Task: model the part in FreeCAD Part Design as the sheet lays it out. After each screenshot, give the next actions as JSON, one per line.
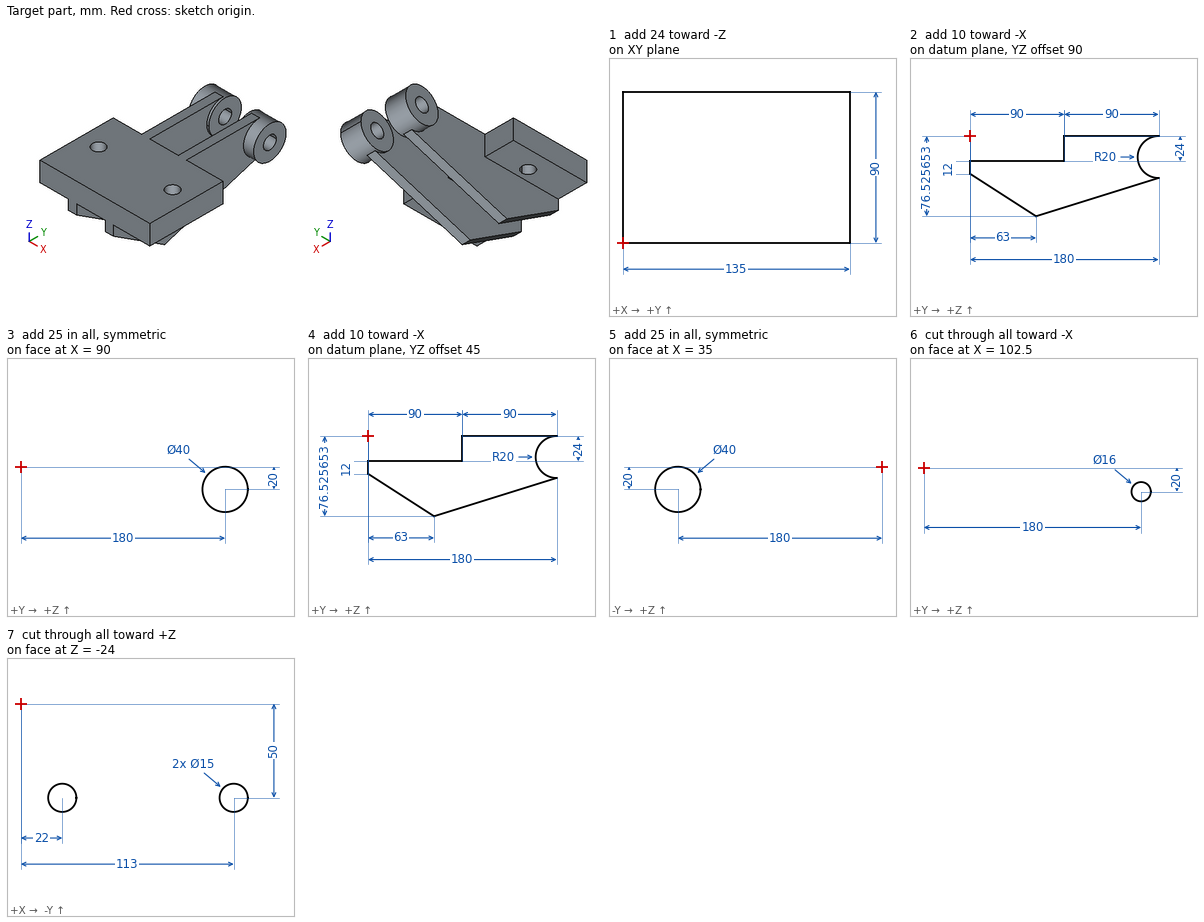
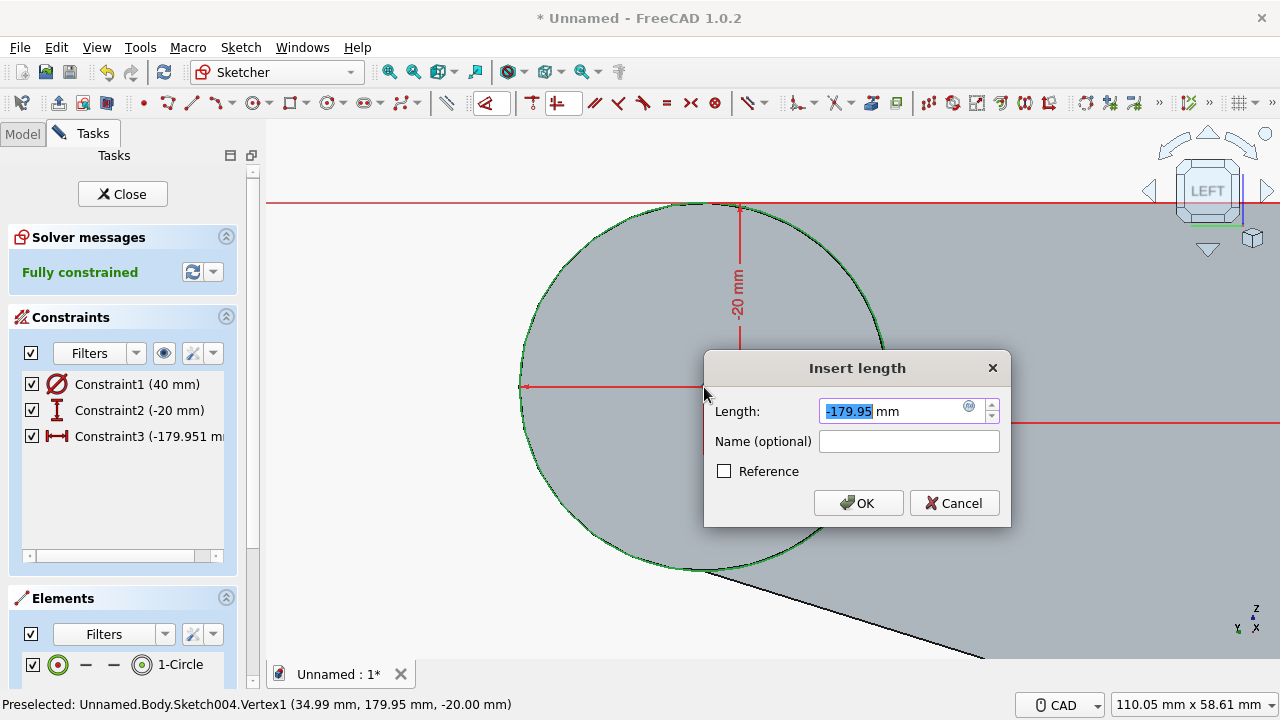
{"action": "type", "text": "-180"}
{"action": "key", "text": "Return"}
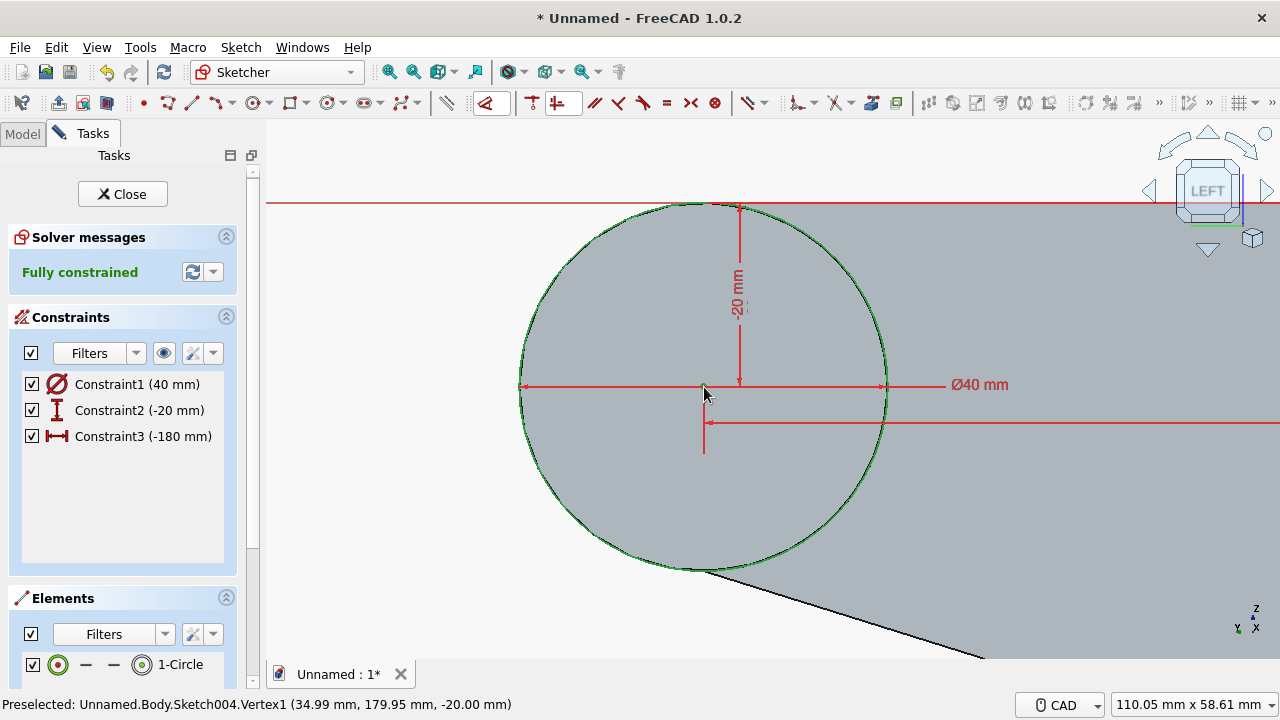
{"action": "left_click", "coordinate": [123, 194]}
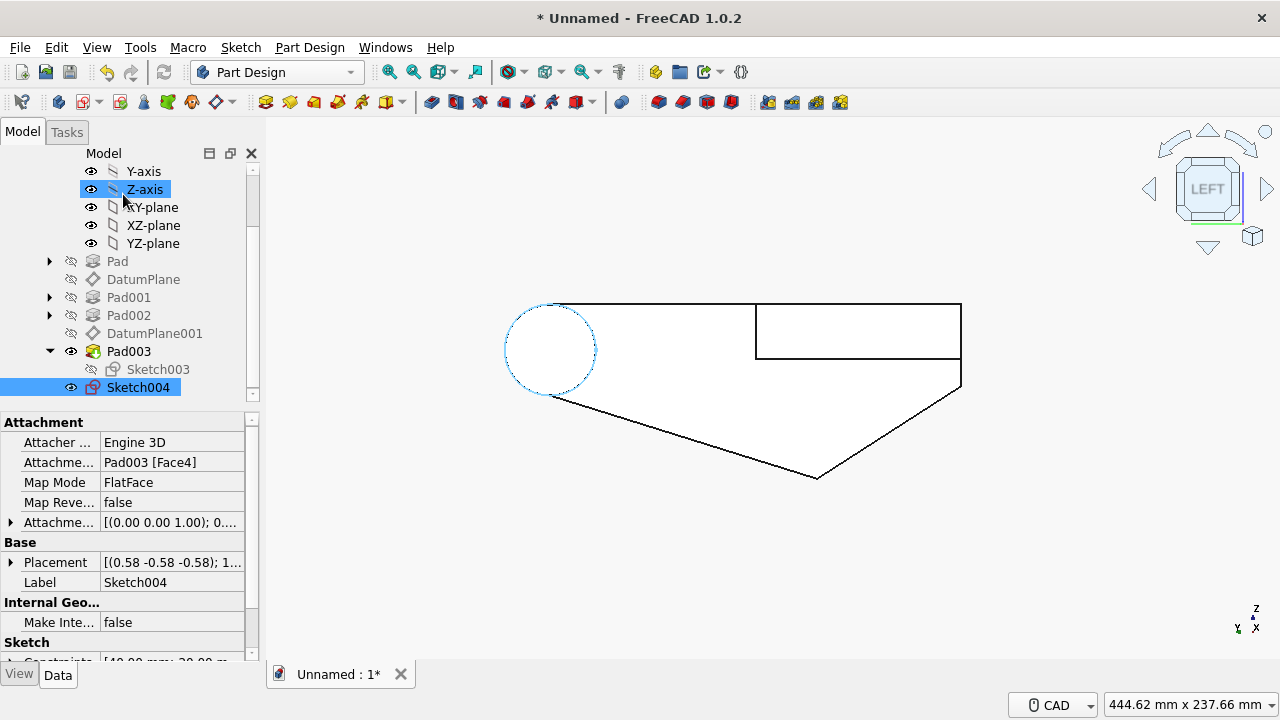
{"action": "left_click", "coordinate": [266, 102]}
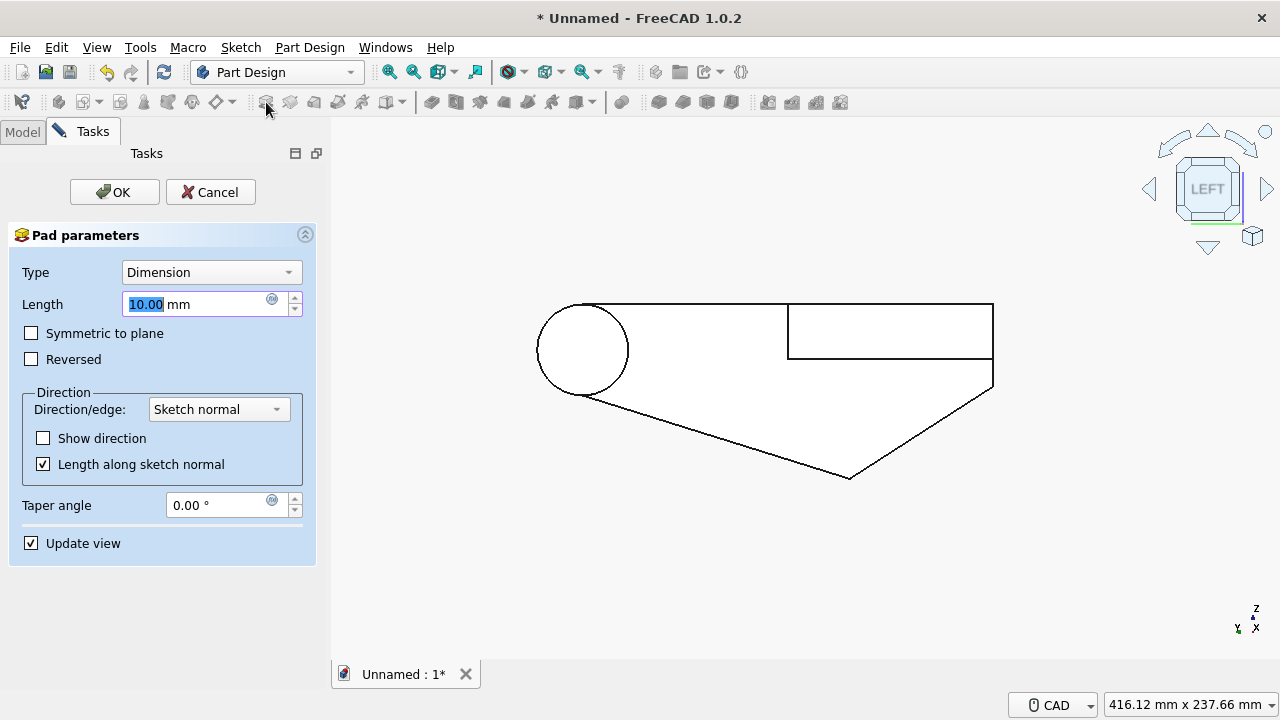
{"action": "type", "text": "25"}
{"action": "key", "text": "Tab"}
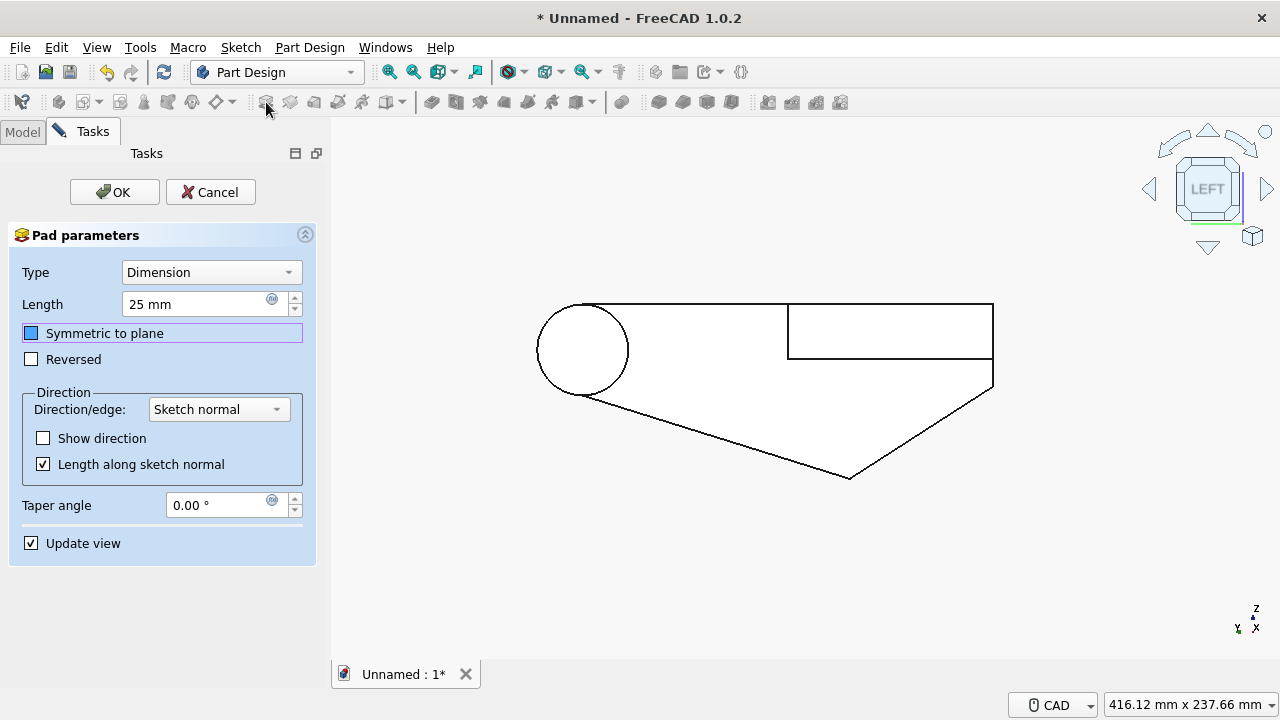
{"action": "left_click", "coordinate": [30, 333]}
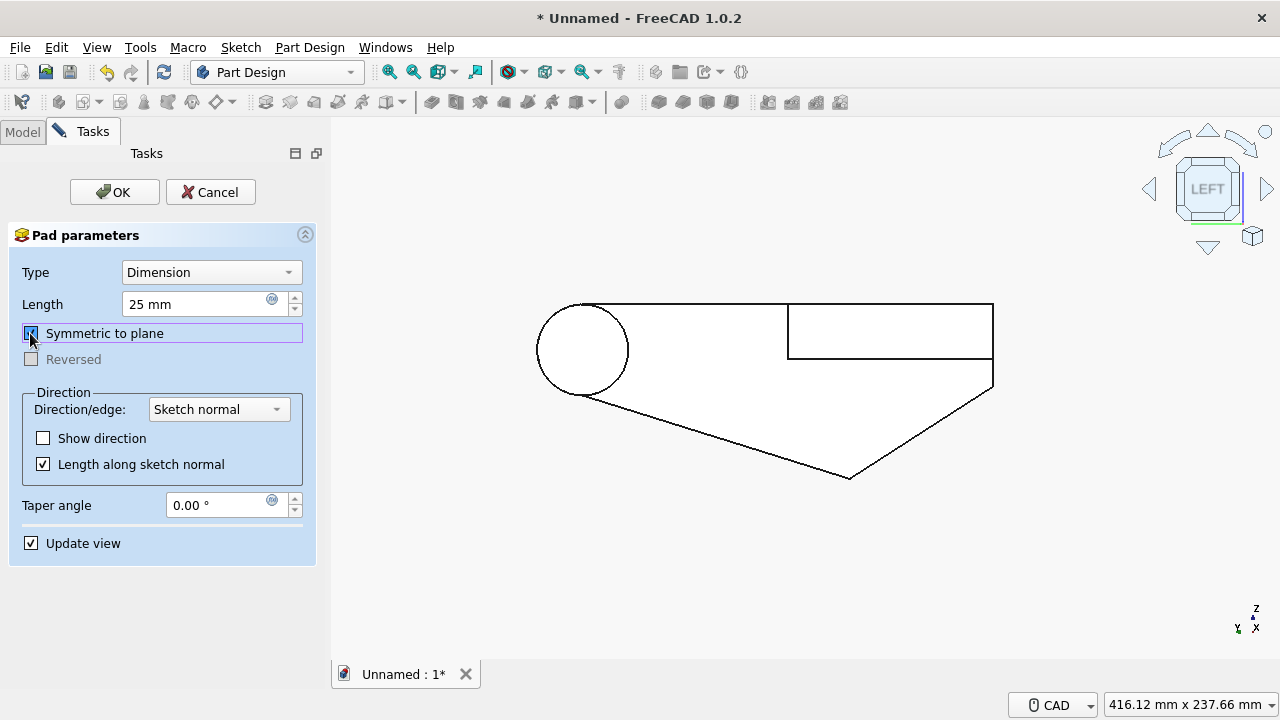
{"action": "left_click", "coordinate": [115, 192]}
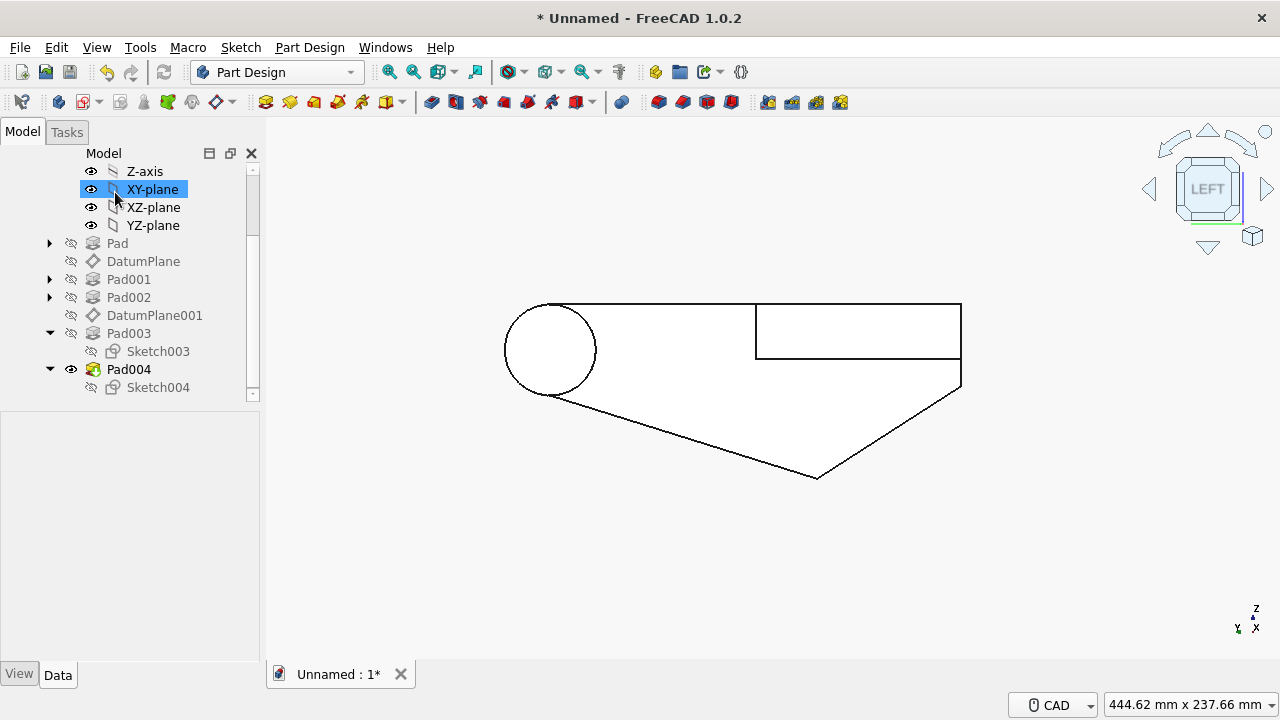
{"action": "left_click", "coordinate": [390, 72]}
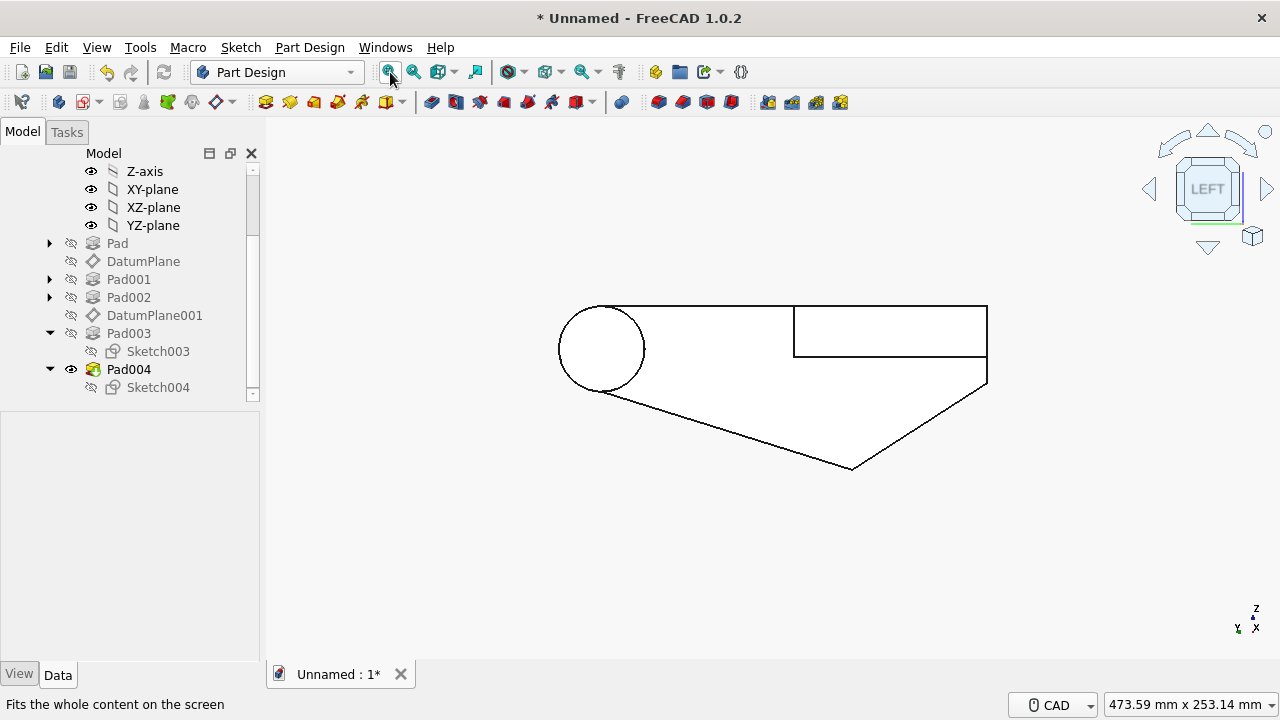
{"action": "key", "text": "0"}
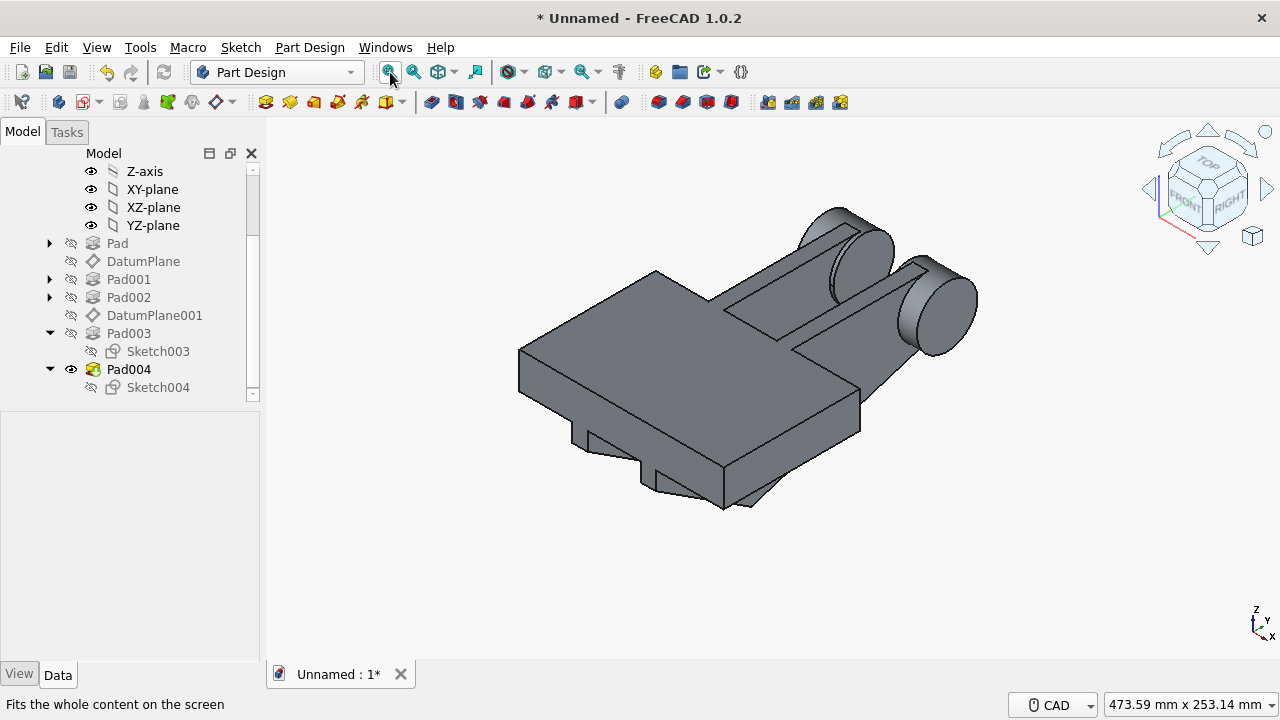
{"action": "left_click", "coordinate": [947, 316]}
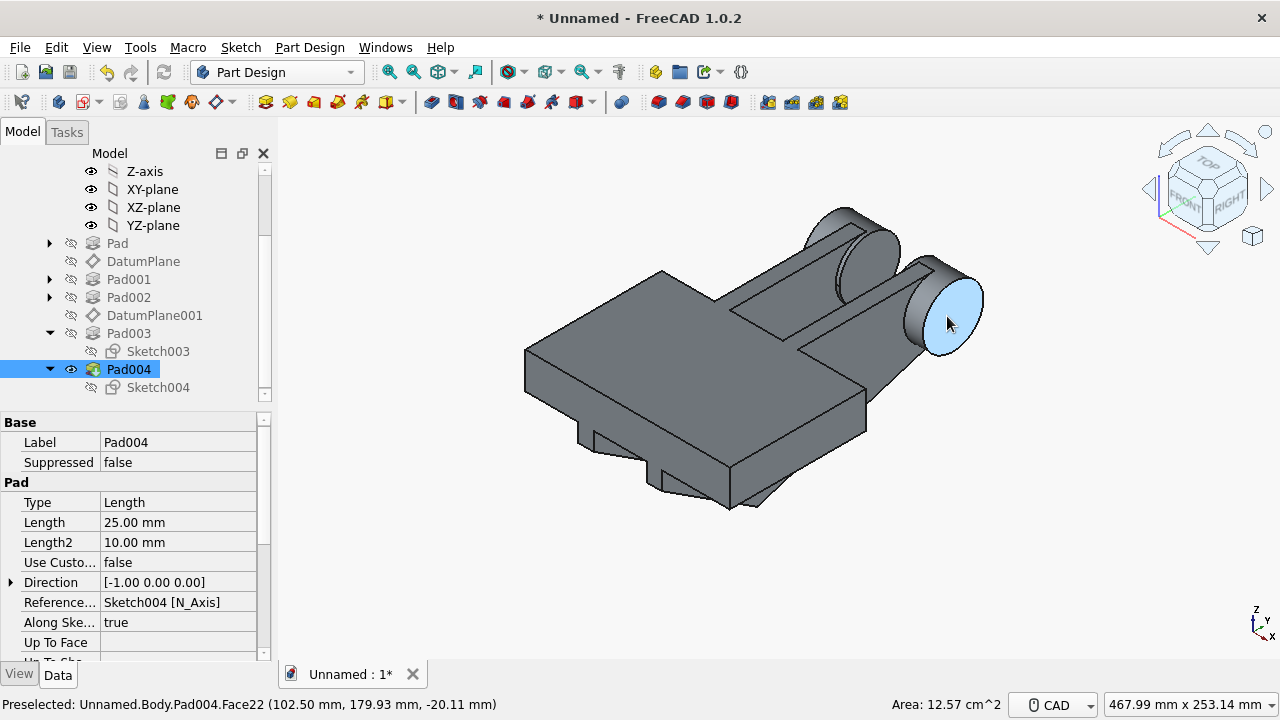
{"action": "left_click", "coordinate": [84, 102]}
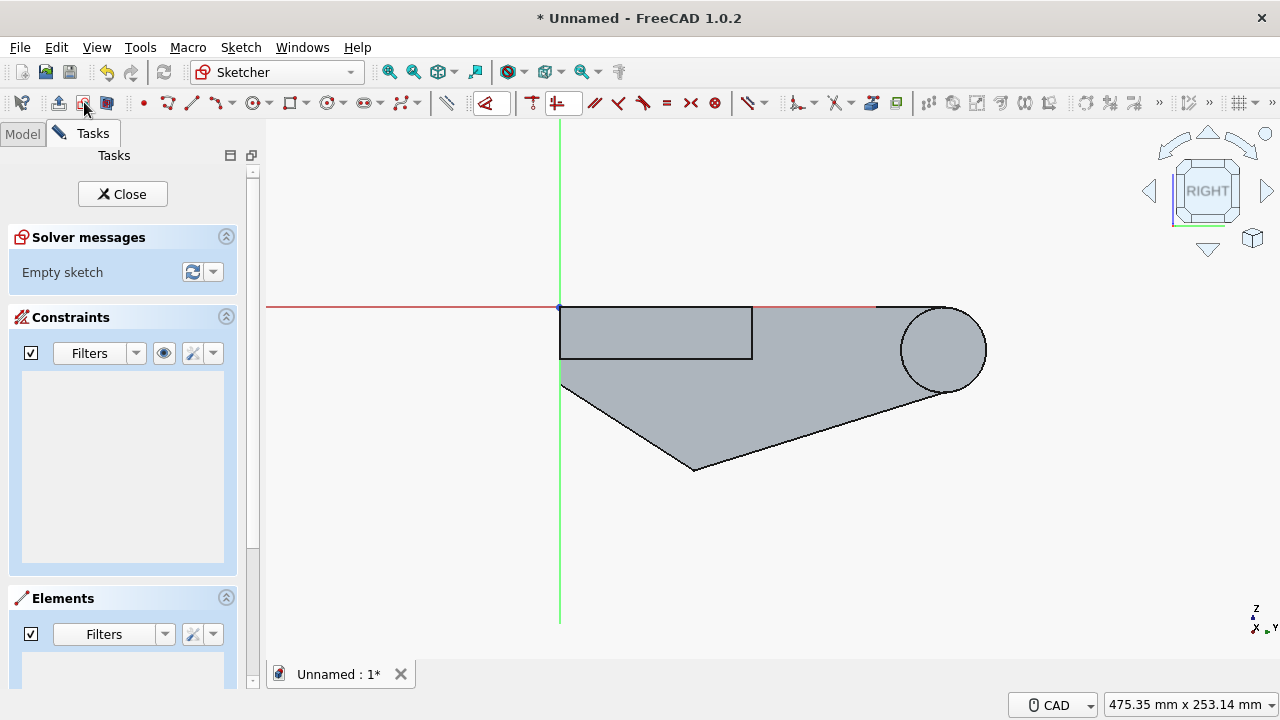
{"action": "key", "text": "q s"}